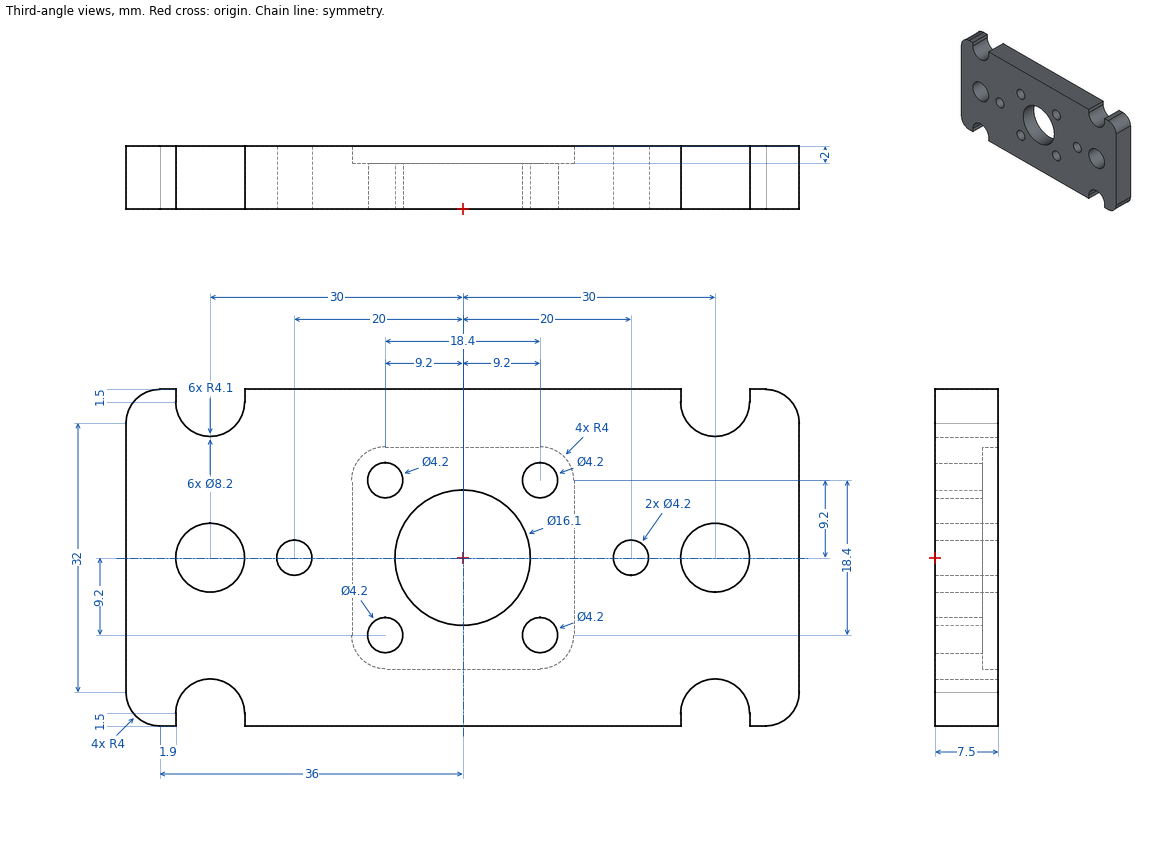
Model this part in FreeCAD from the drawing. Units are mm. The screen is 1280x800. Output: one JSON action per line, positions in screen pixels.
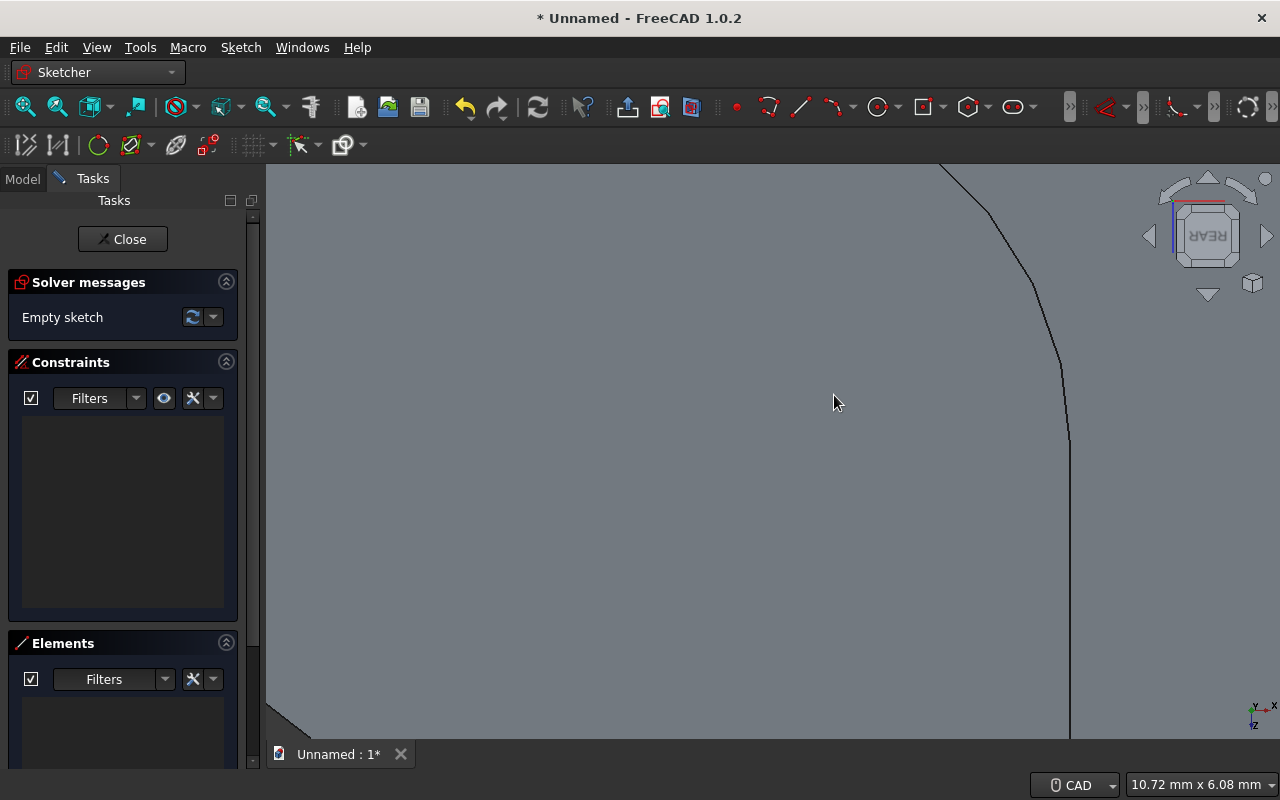
{"action": "left_click", "coordinate": [878, 108]}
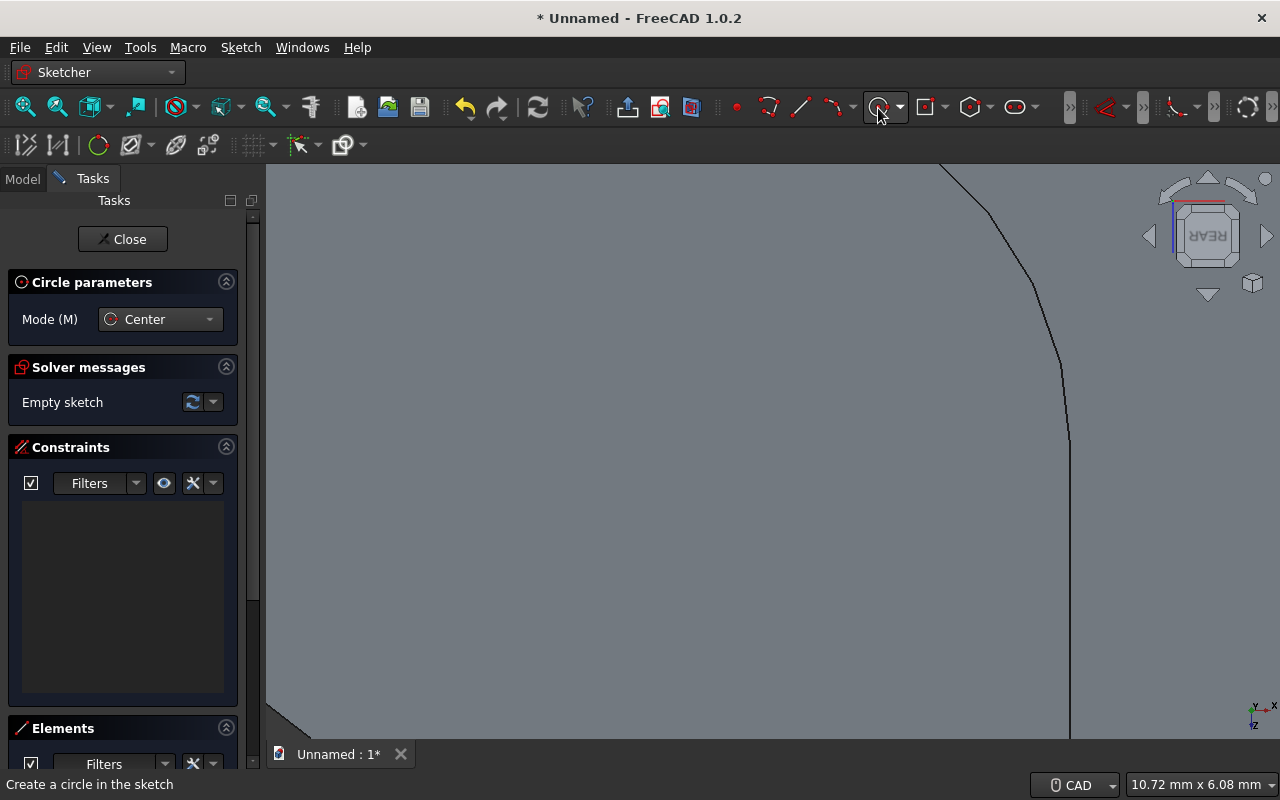
{"action": "left_click", "coordinate": [692, 448]}
{"action": "mouse_move", "coordinate": [833, 308]}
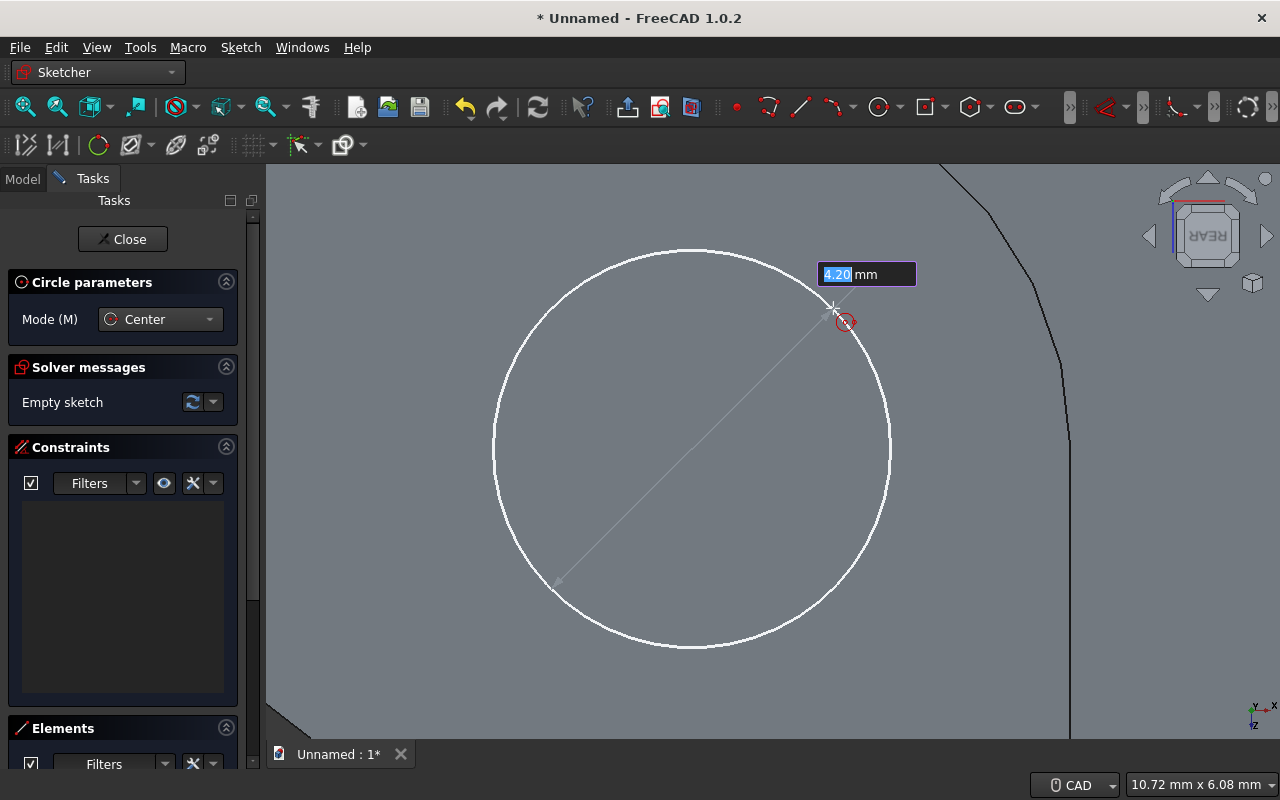
{"action": "type", "text": "4.2"}
{"action": "key", "text": "Return"}
{"action": "key", "text": "Escape"}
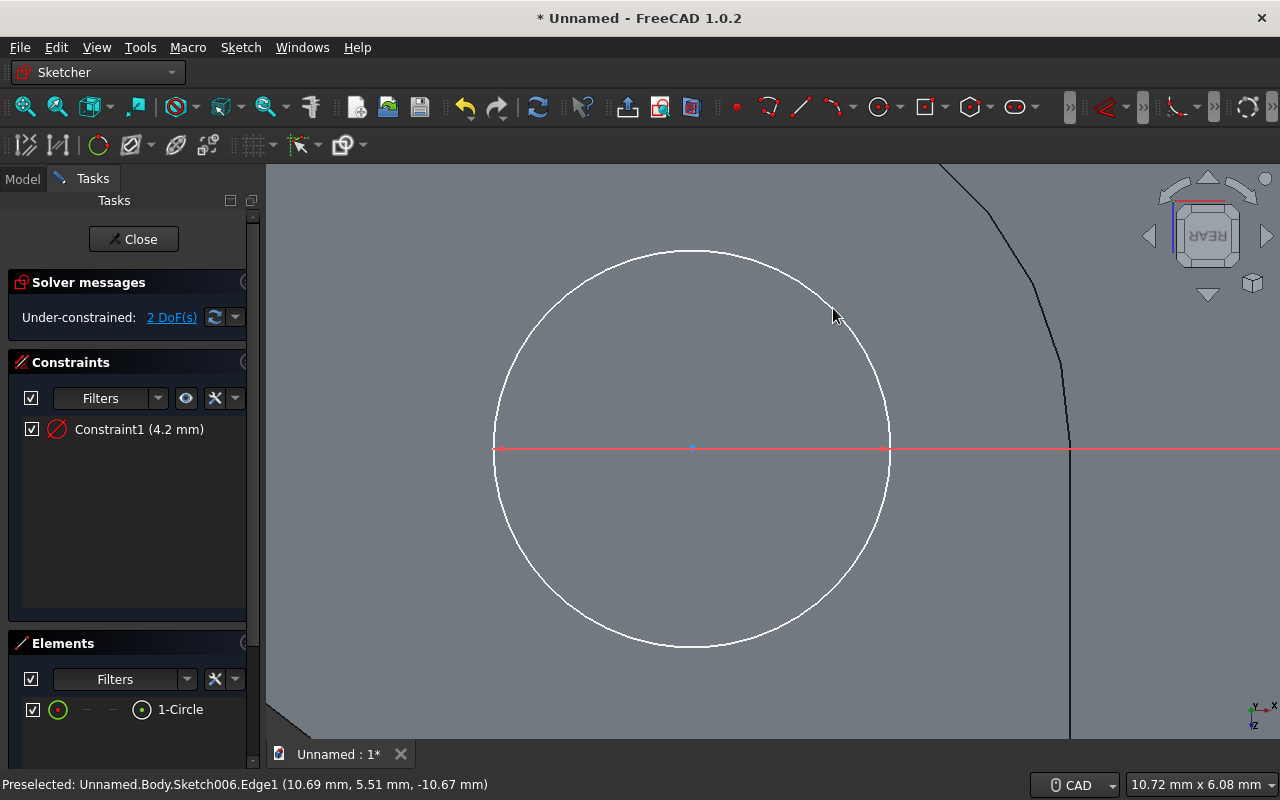
{"action": "left_click", "coordinate": [1106, 108]}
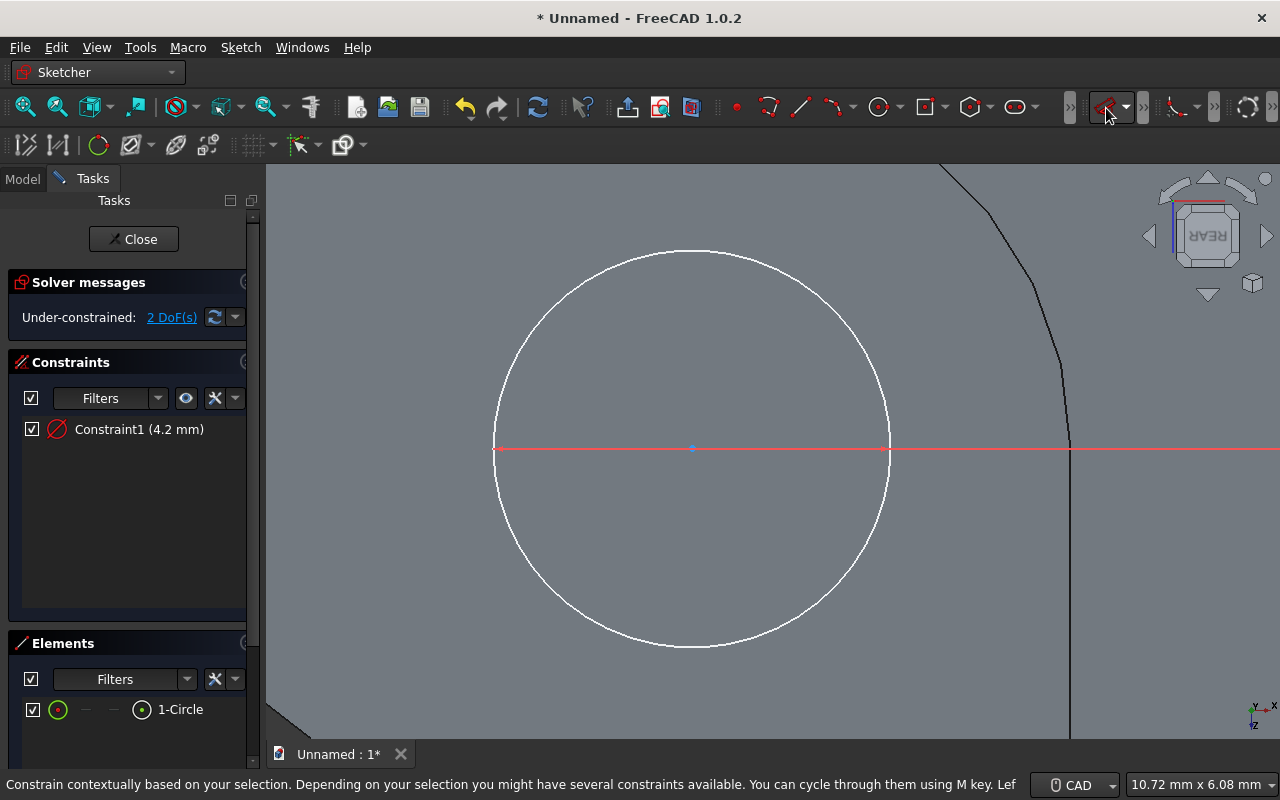
{"action": "left_click", "coordinate": [692, 449]}
{"action": "left_click", "coordinate": [401, 415]}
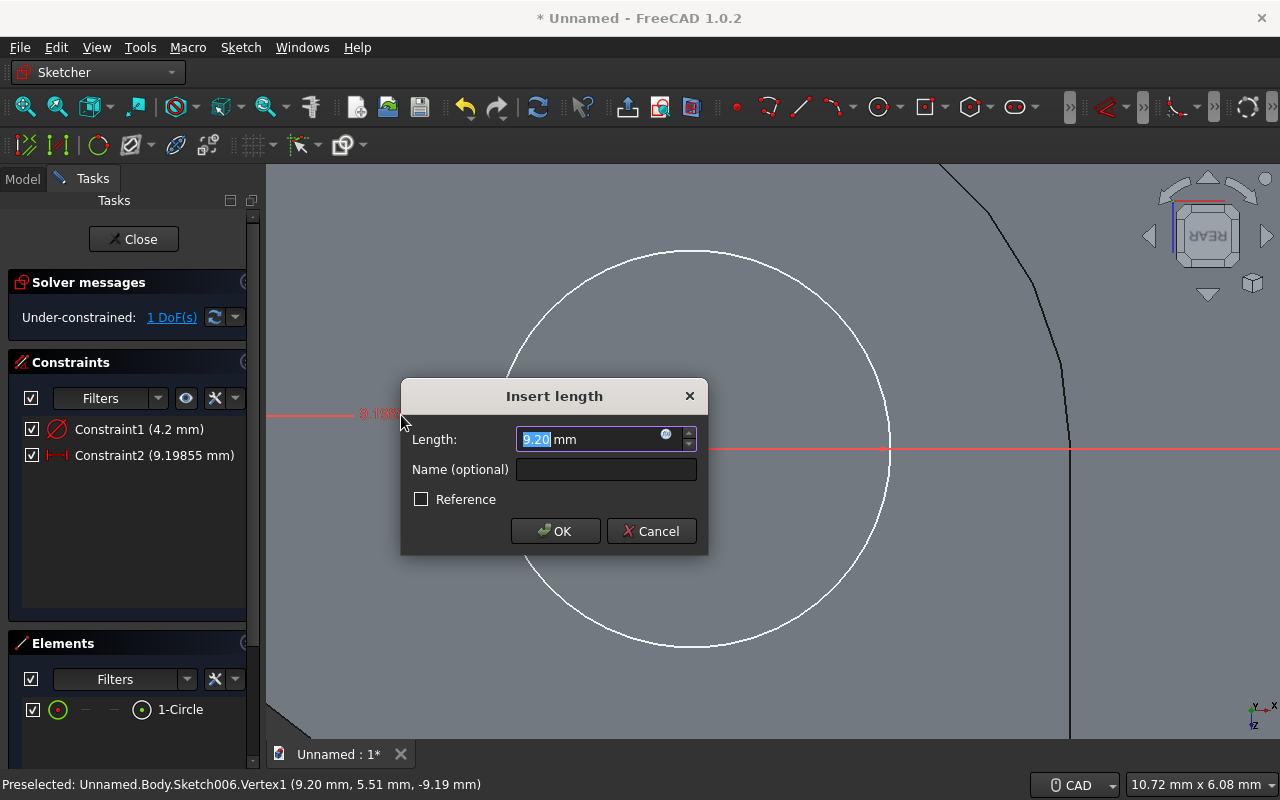
{"action": "type", "text": "9.2"}
{"action": "key", "text": "Return"}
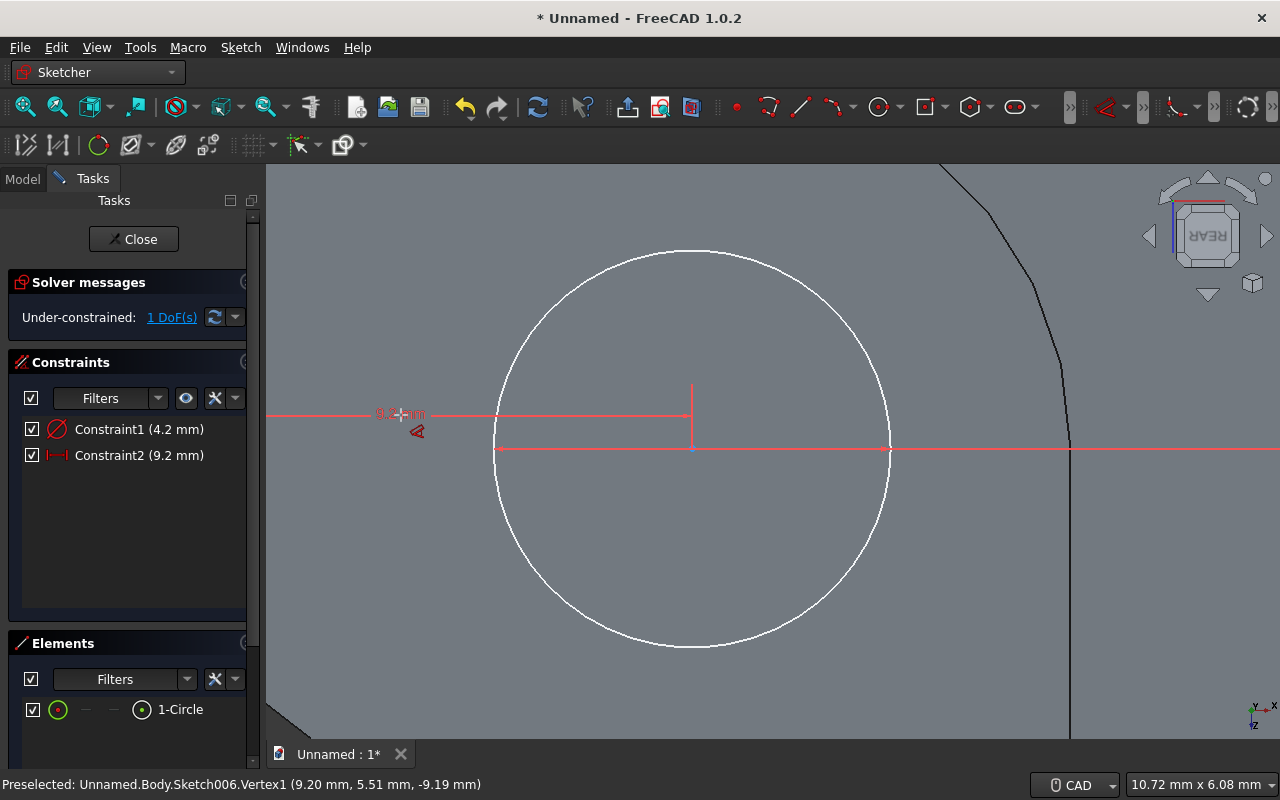
{"action": "left_click", "coordinate": [692, 449]}
{"action": "left_click", "coordinate": [726, 580]}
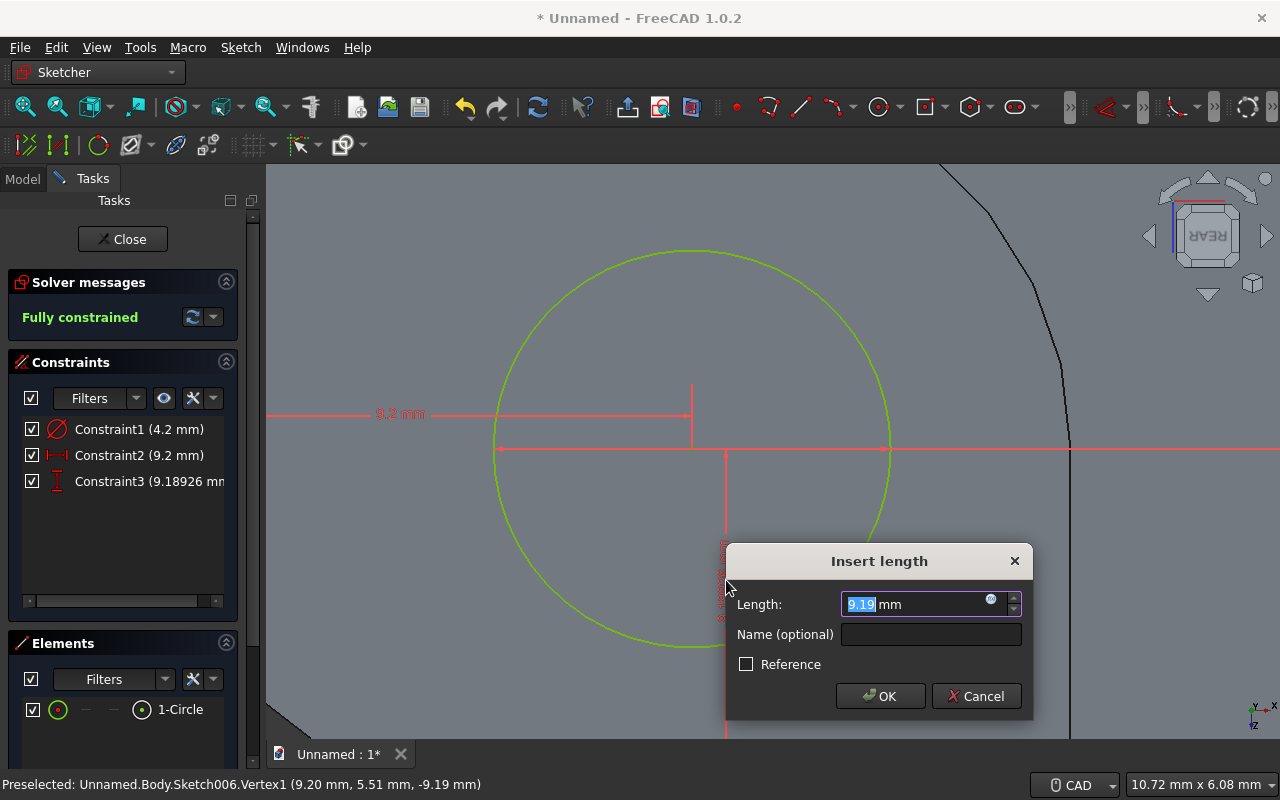
{"action": "type", "text": "9.2"}
{"action": "key", "text": "Return"}
{"action": "key", "text": "Escape"}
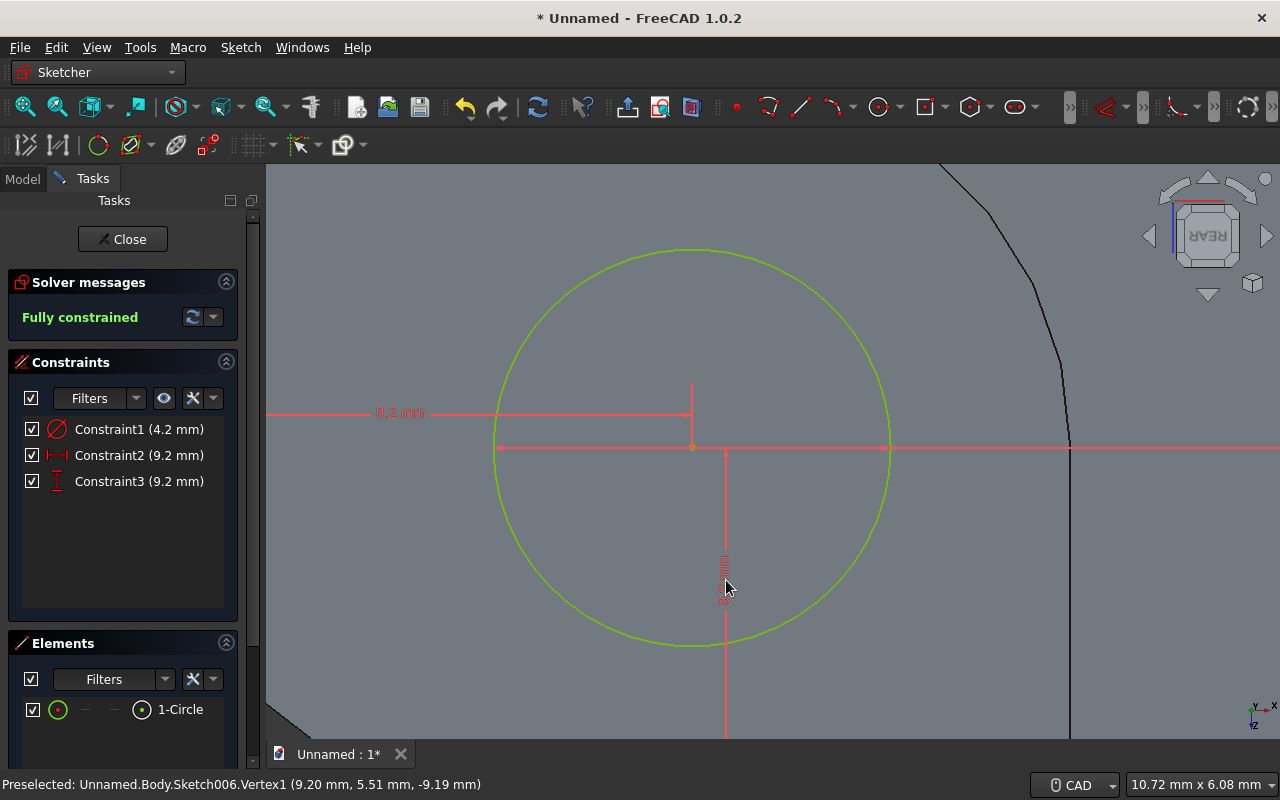
{"action": "left_click", "coordinate": [123, 239]}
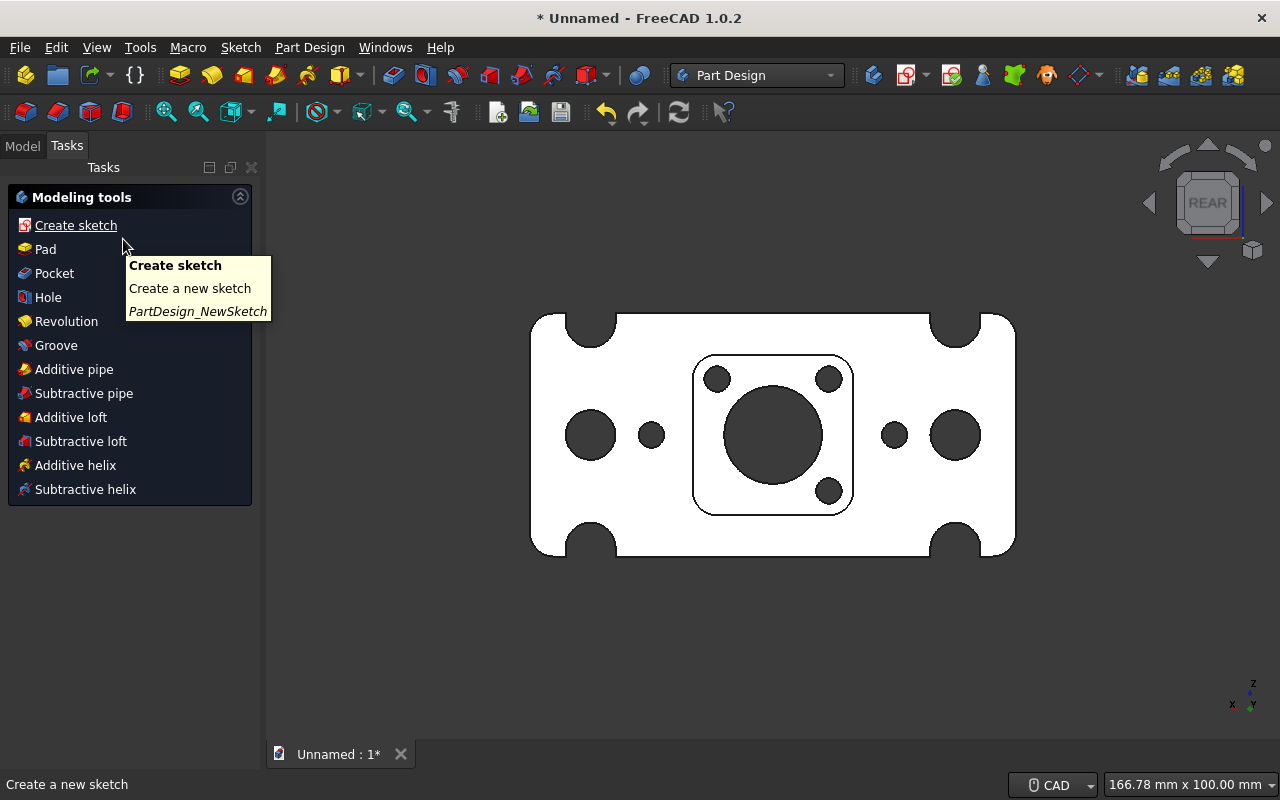
{"action": "left_click", "coordinate": [394, 76]}